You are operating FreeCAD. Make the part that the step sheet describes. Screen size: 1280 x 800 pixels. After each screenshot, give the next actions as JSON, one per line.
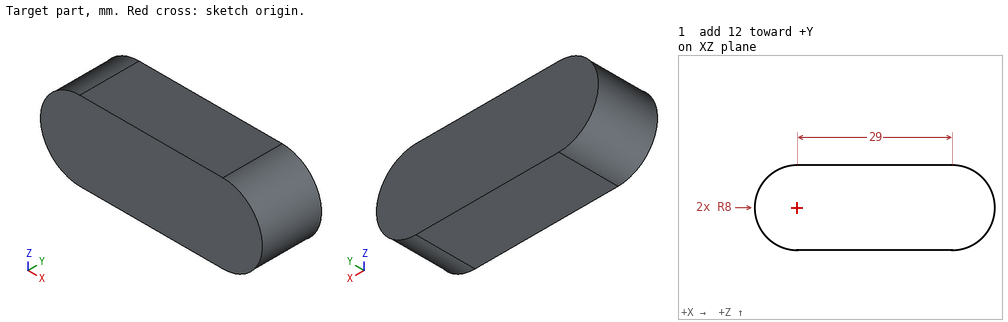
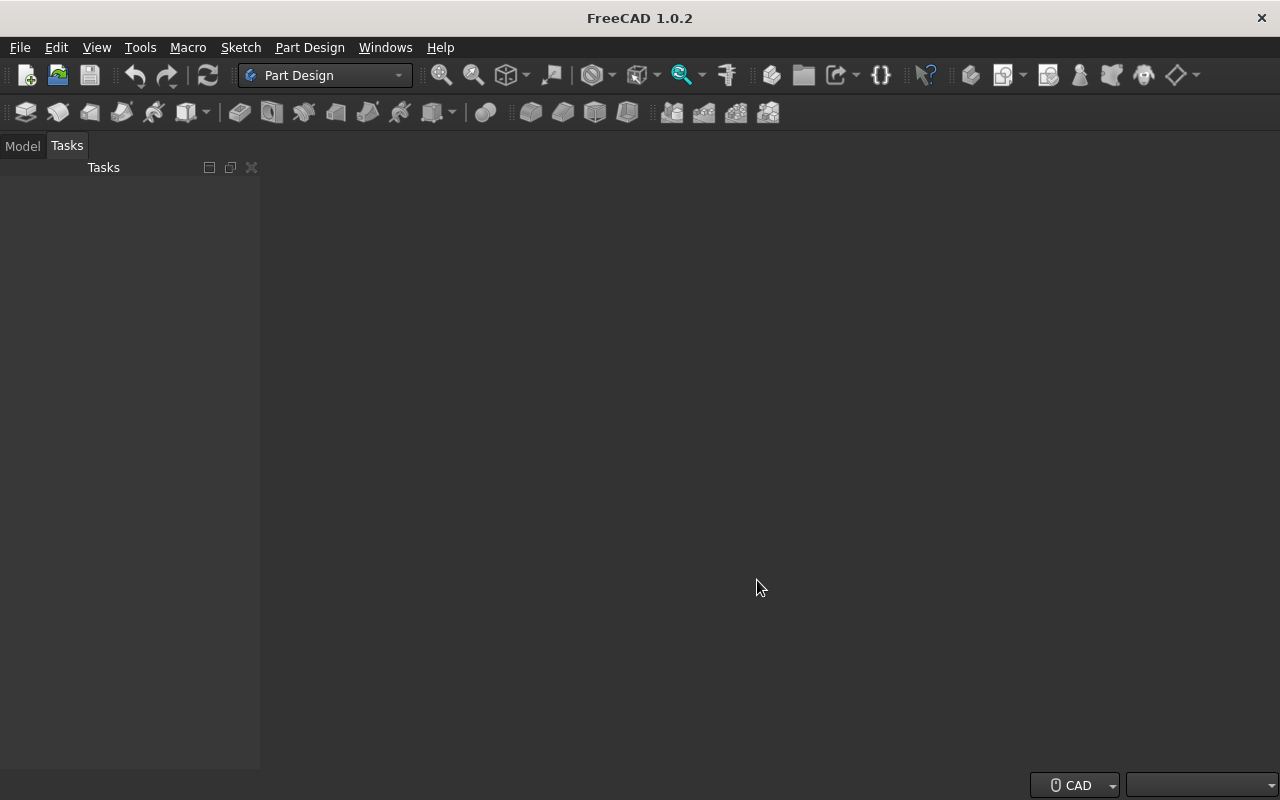
{"action": "left_click", "coordinate": [26, 76]}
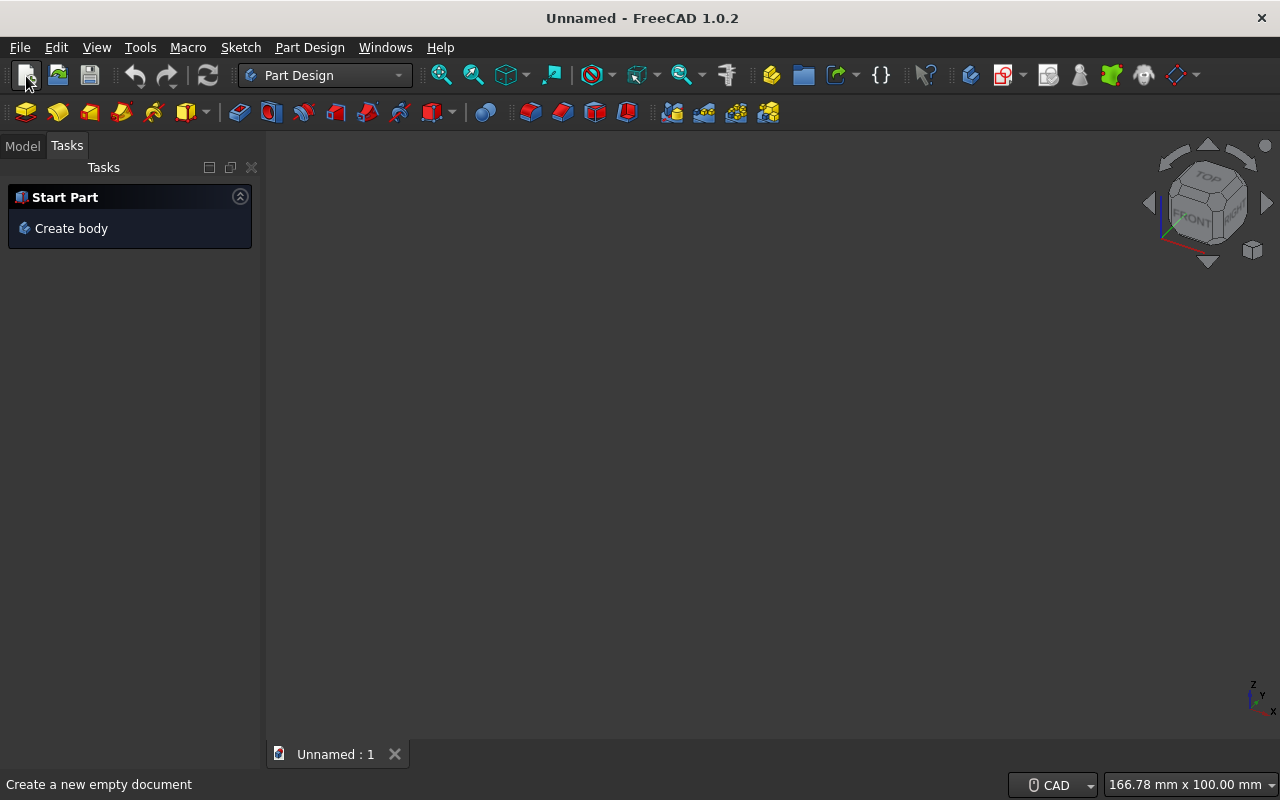
{"action": "left_click", "coordinate": [1004, 76]}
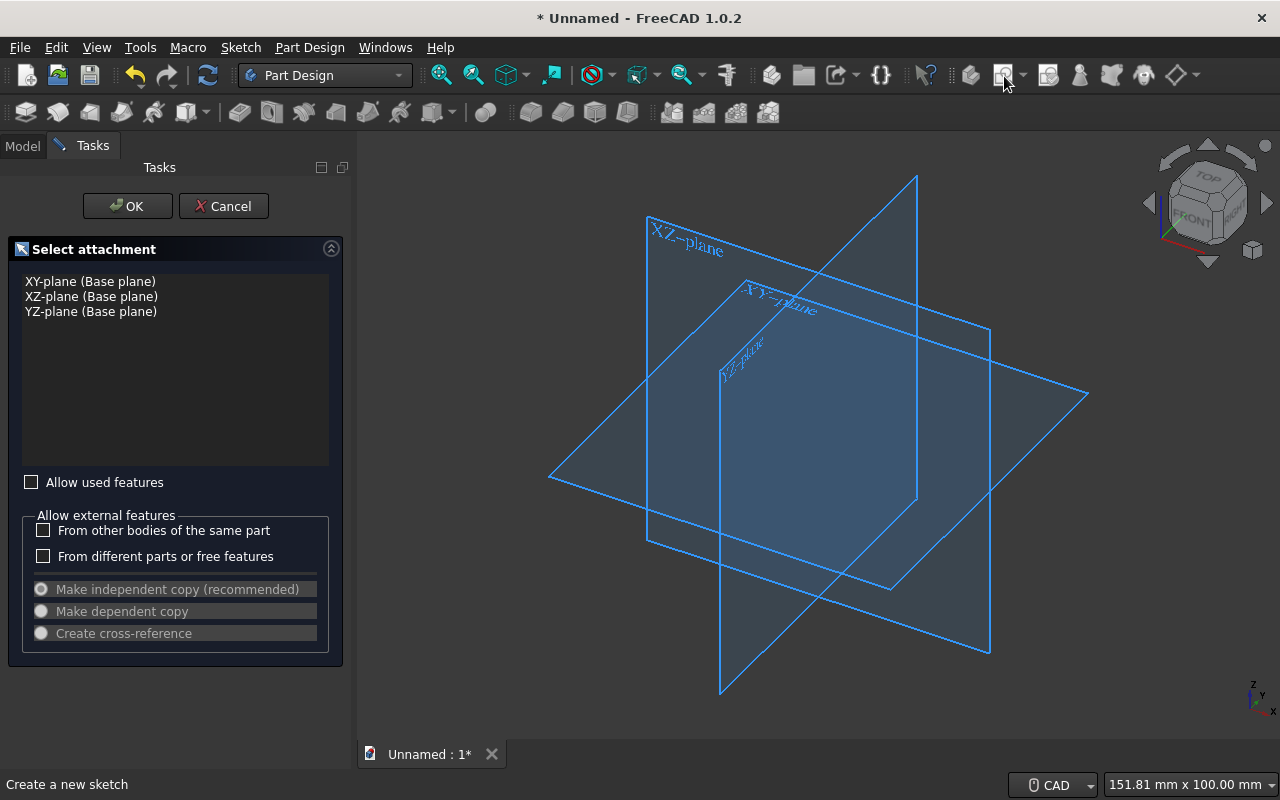
{"action": "left_click", "coordinate": [82, 296]}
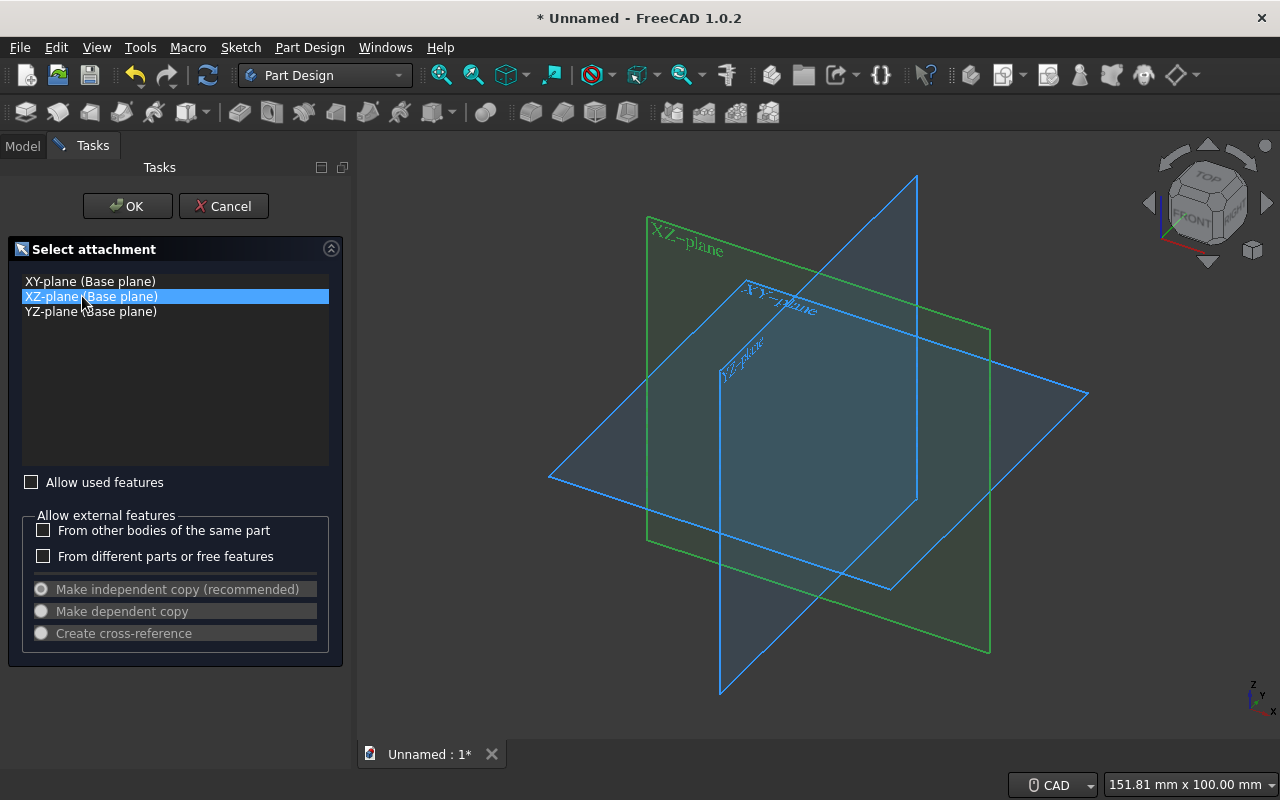
{"action": "left_click", "coordinate": [128, 206]}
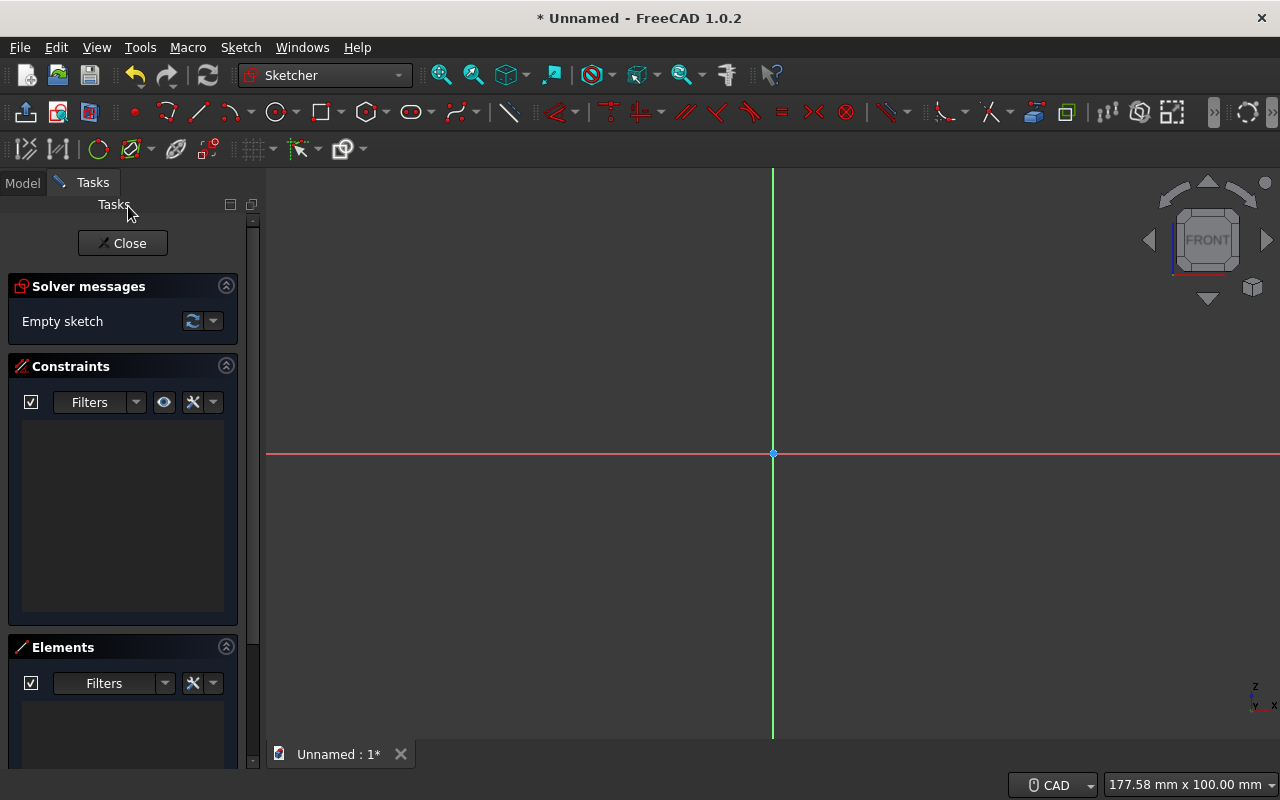
{"action": "scroll", "coordinate": [979, 454], "scroll_direction": "up", "scroll_amount": 4}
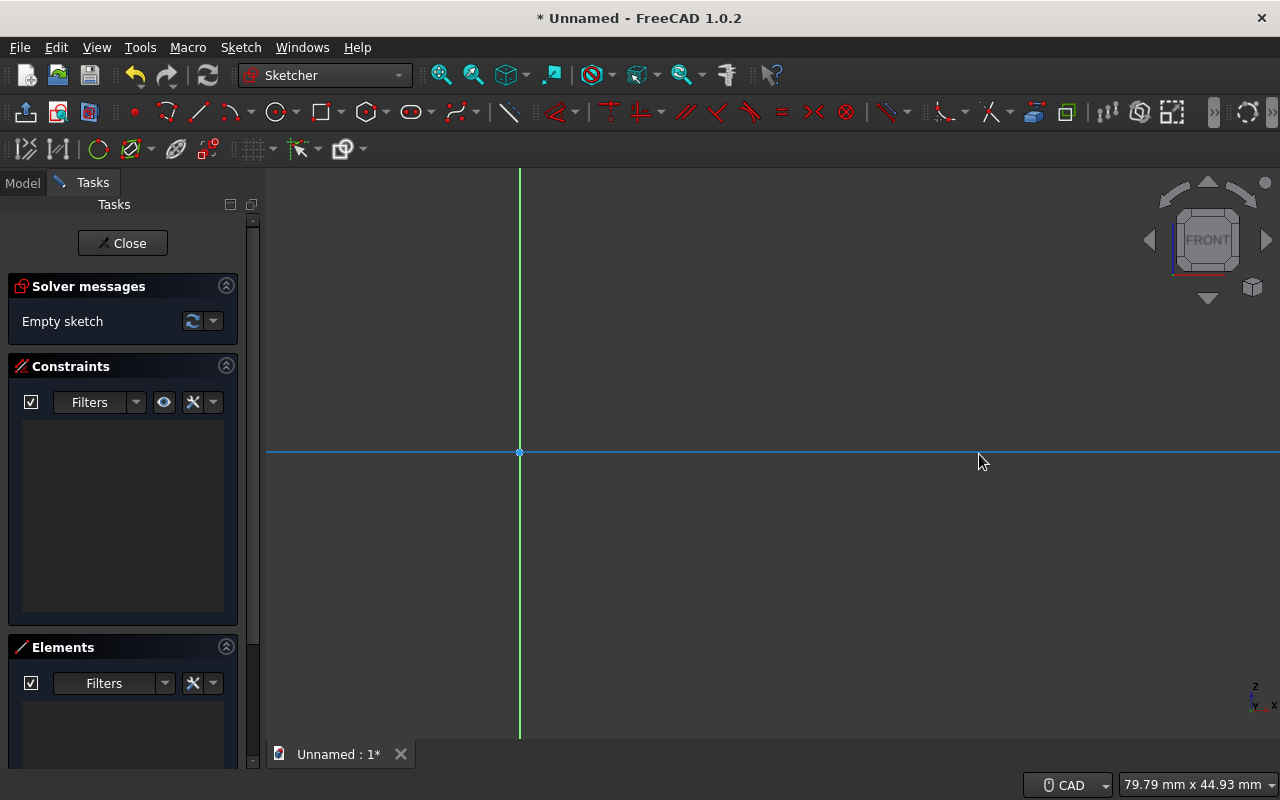
{"action": "left_click", "coordinate": [412, 112]}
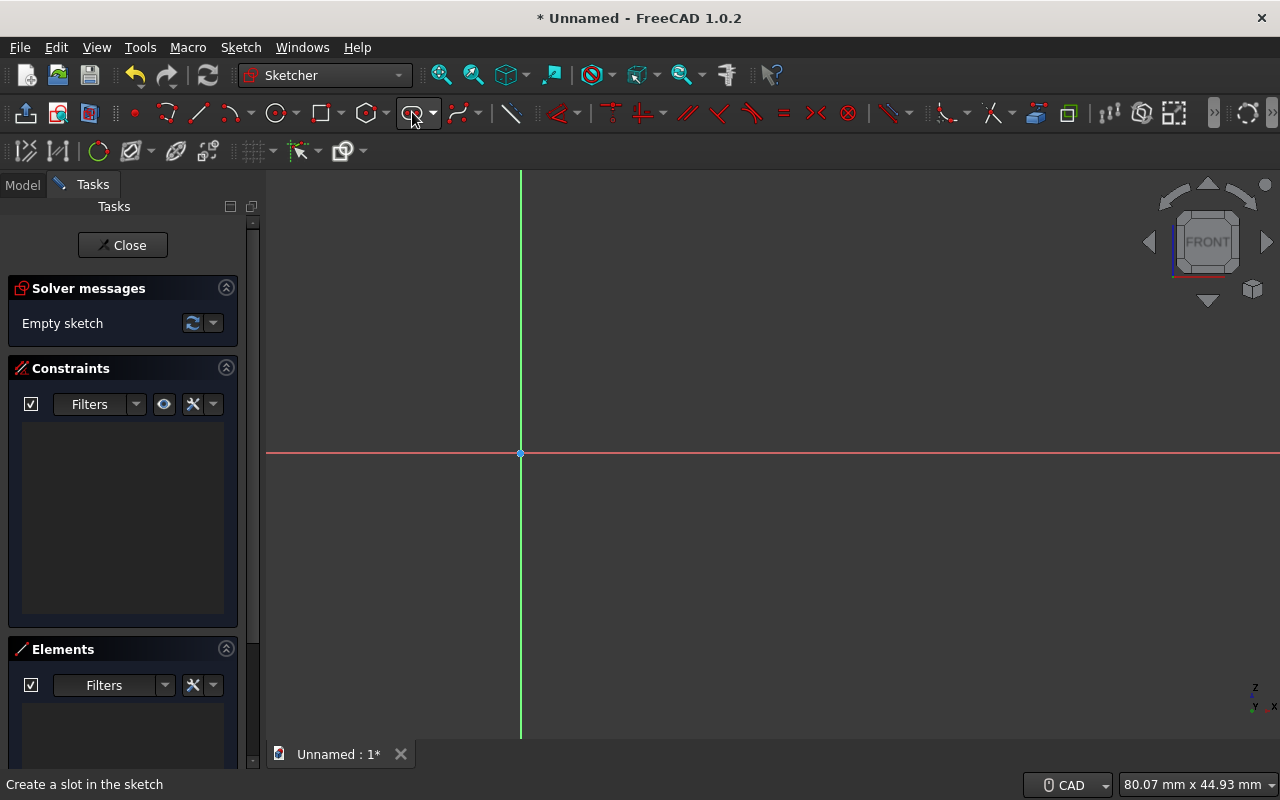
{"action": "left_click", "coordinate": [521, 453]}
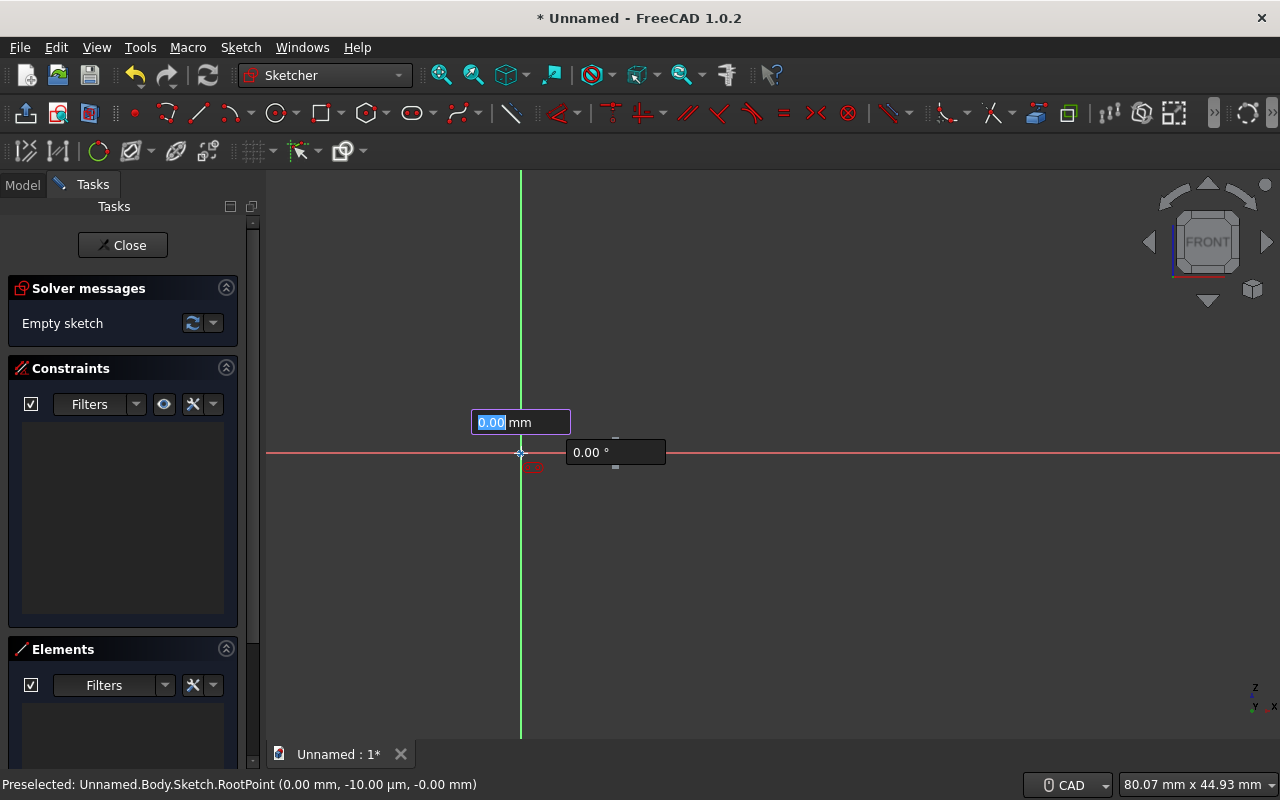
{"action": "left_click", "coordinate": [888, 444]}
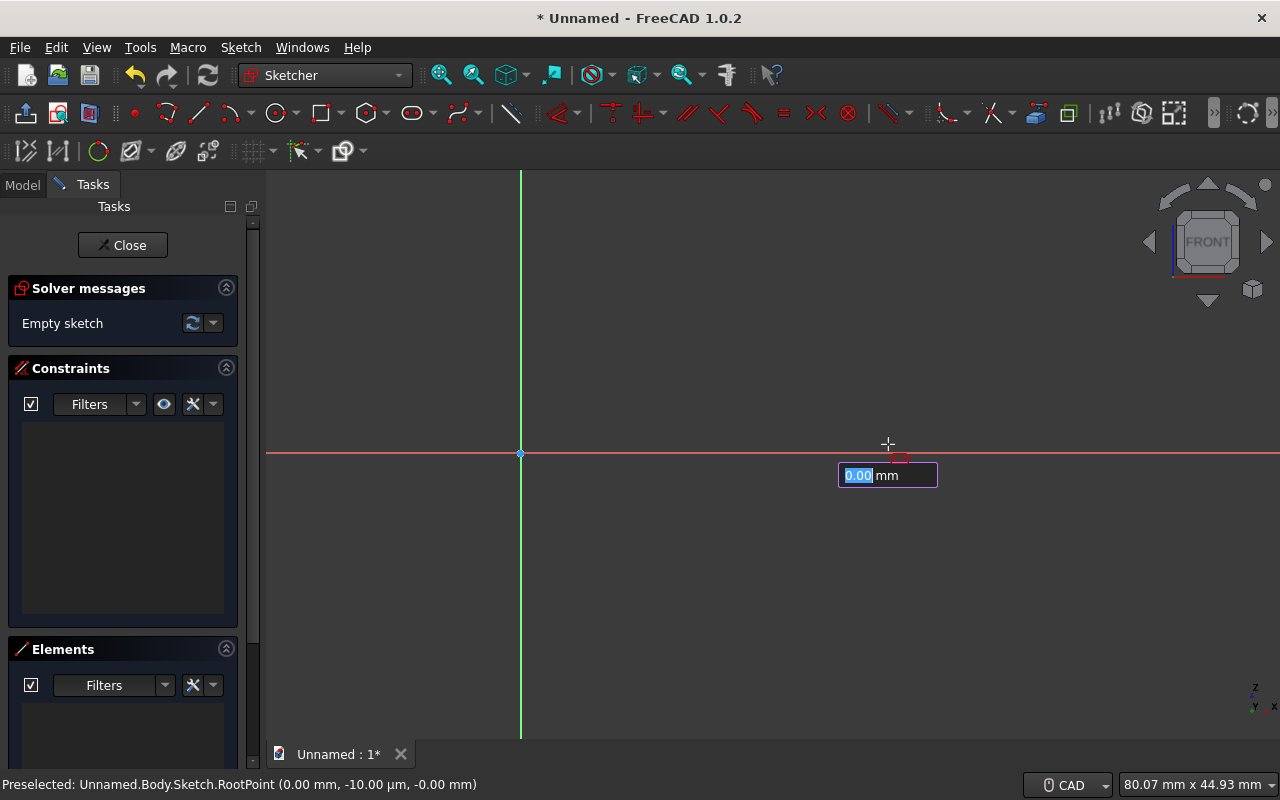
{"action": "left_click", "coordinate": [704, 555]}
{"action": "key", "text": "Escape"}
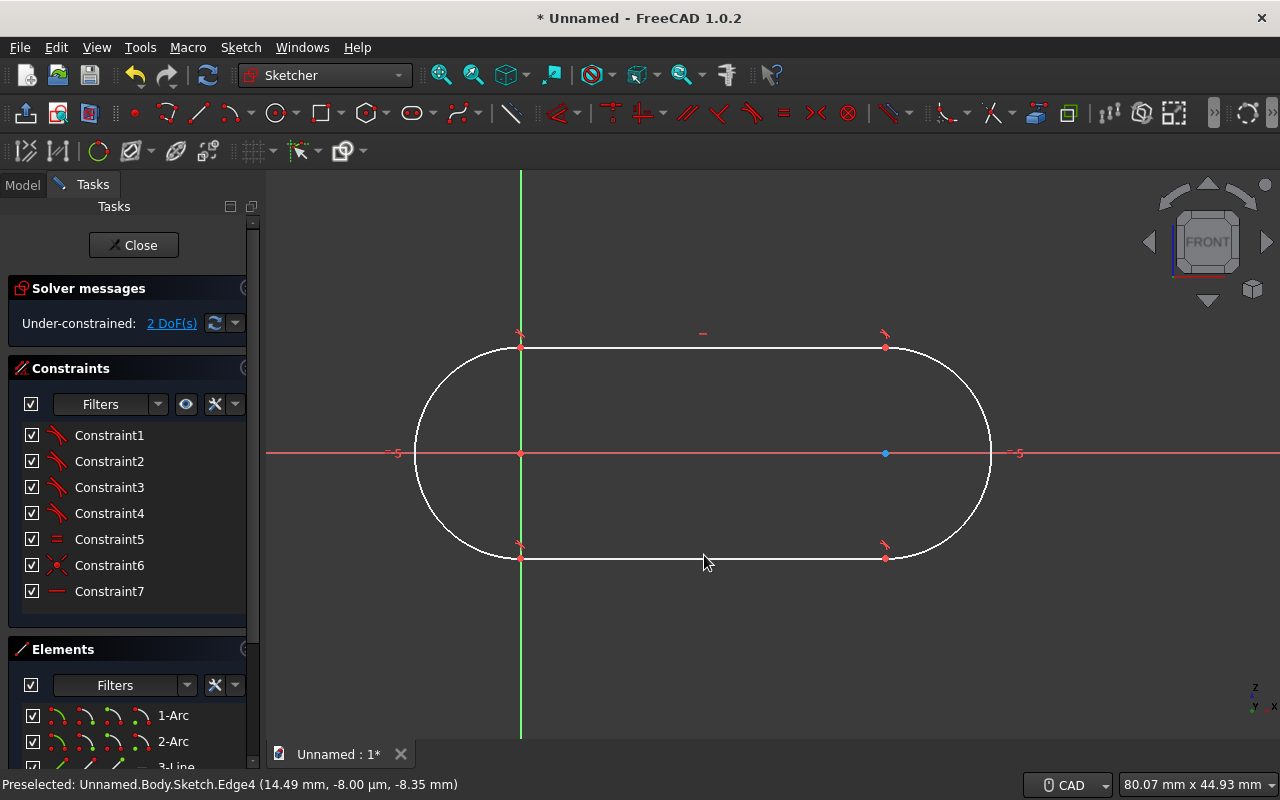
{"action": "left_click", "coordinate": [558, 114]}